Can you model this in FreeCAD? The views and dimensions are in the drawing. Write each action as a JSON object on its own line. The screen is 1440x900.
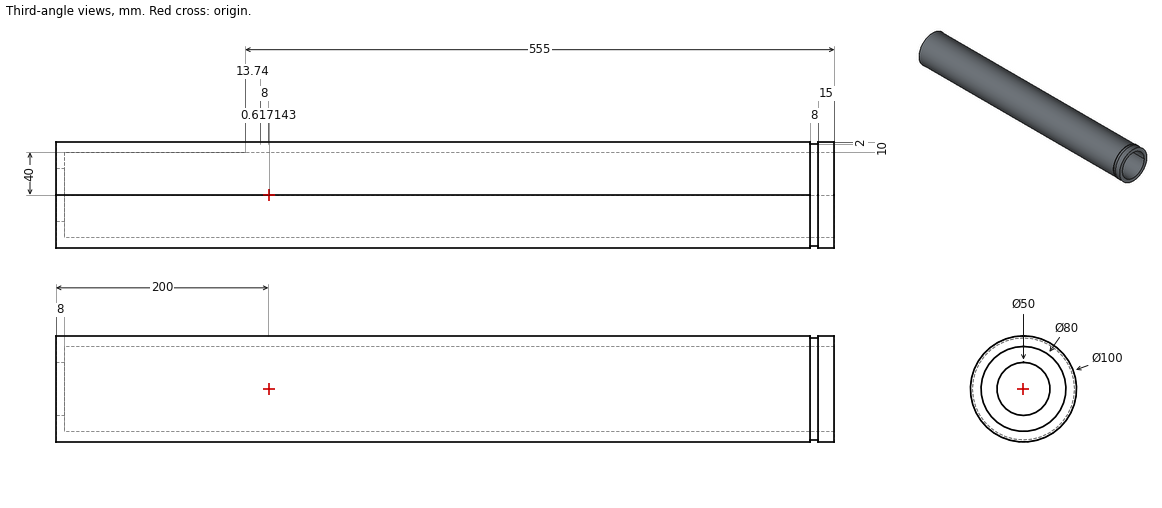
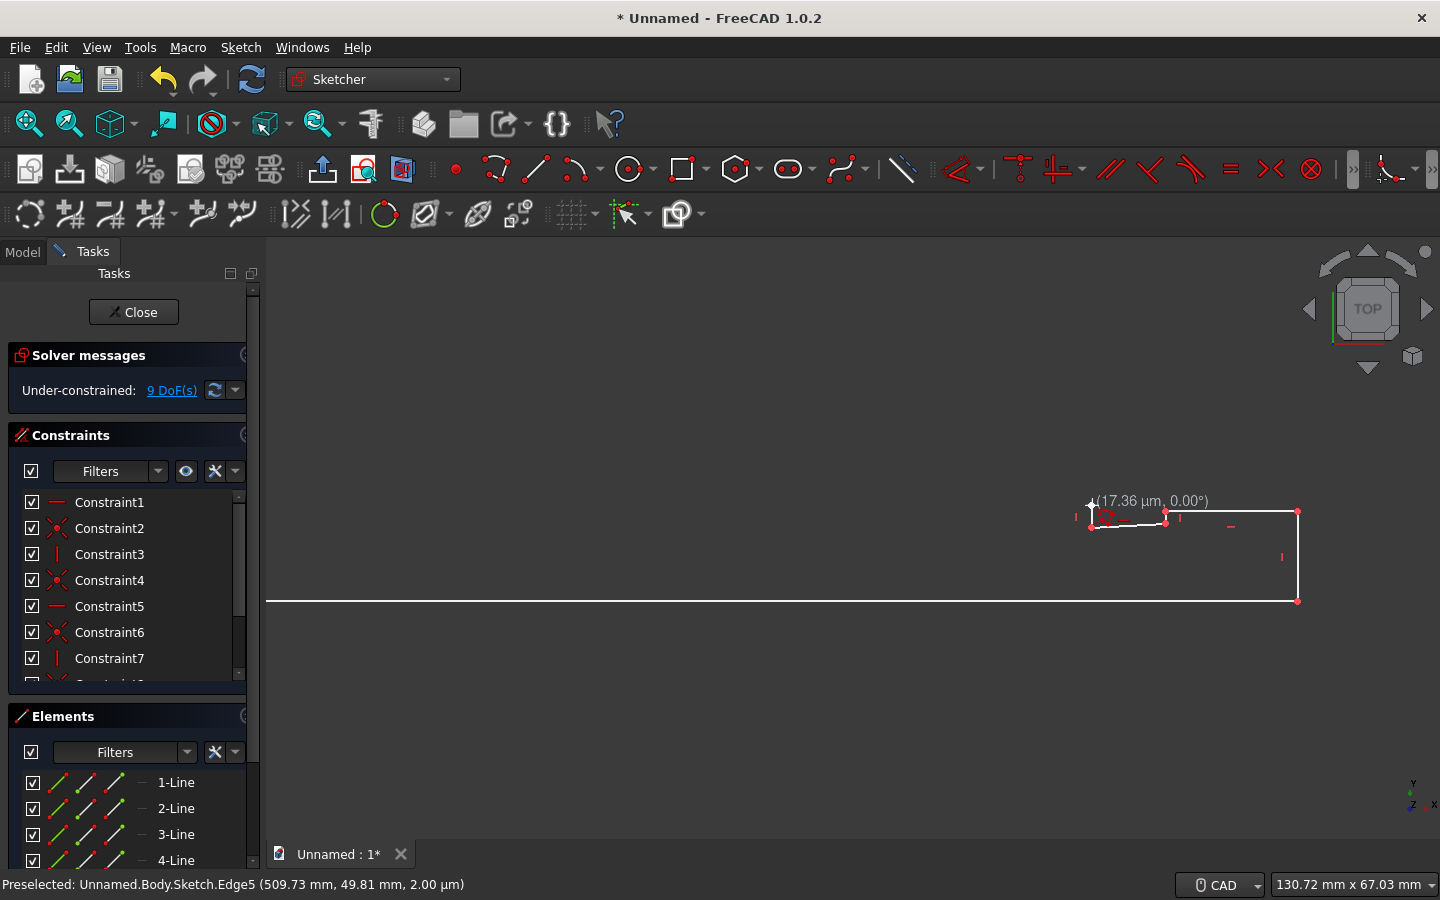
{"action": "scroll", "coordinate": [1094, 508], "scroll_direction": "down", "scroll_amount": 10}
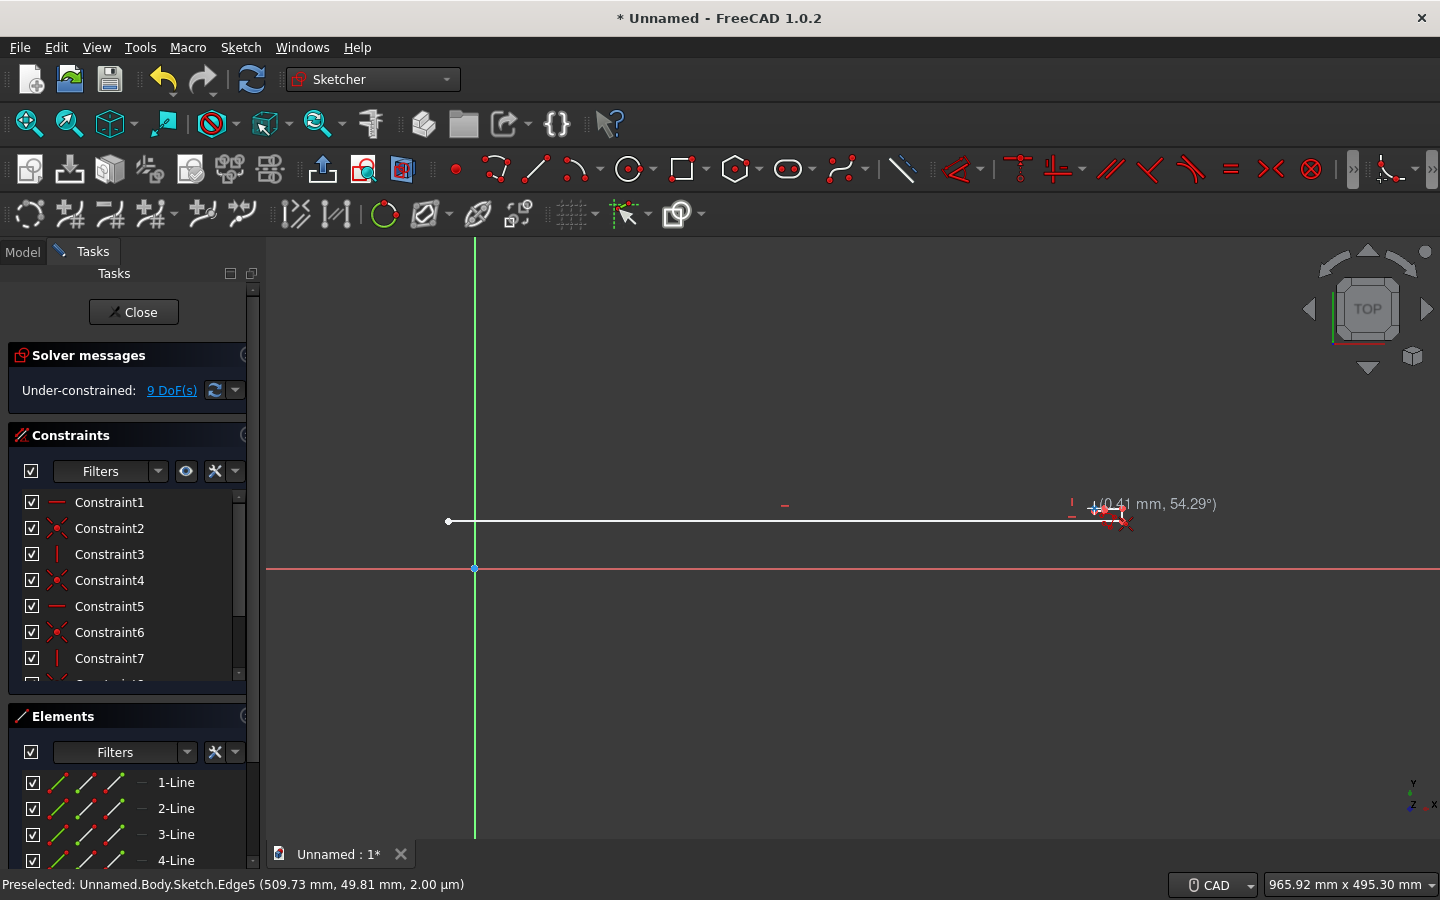
{"action": "scroll", "coordinate": [474, 508], "scroll_direction": "up", "scroll_amount": 16}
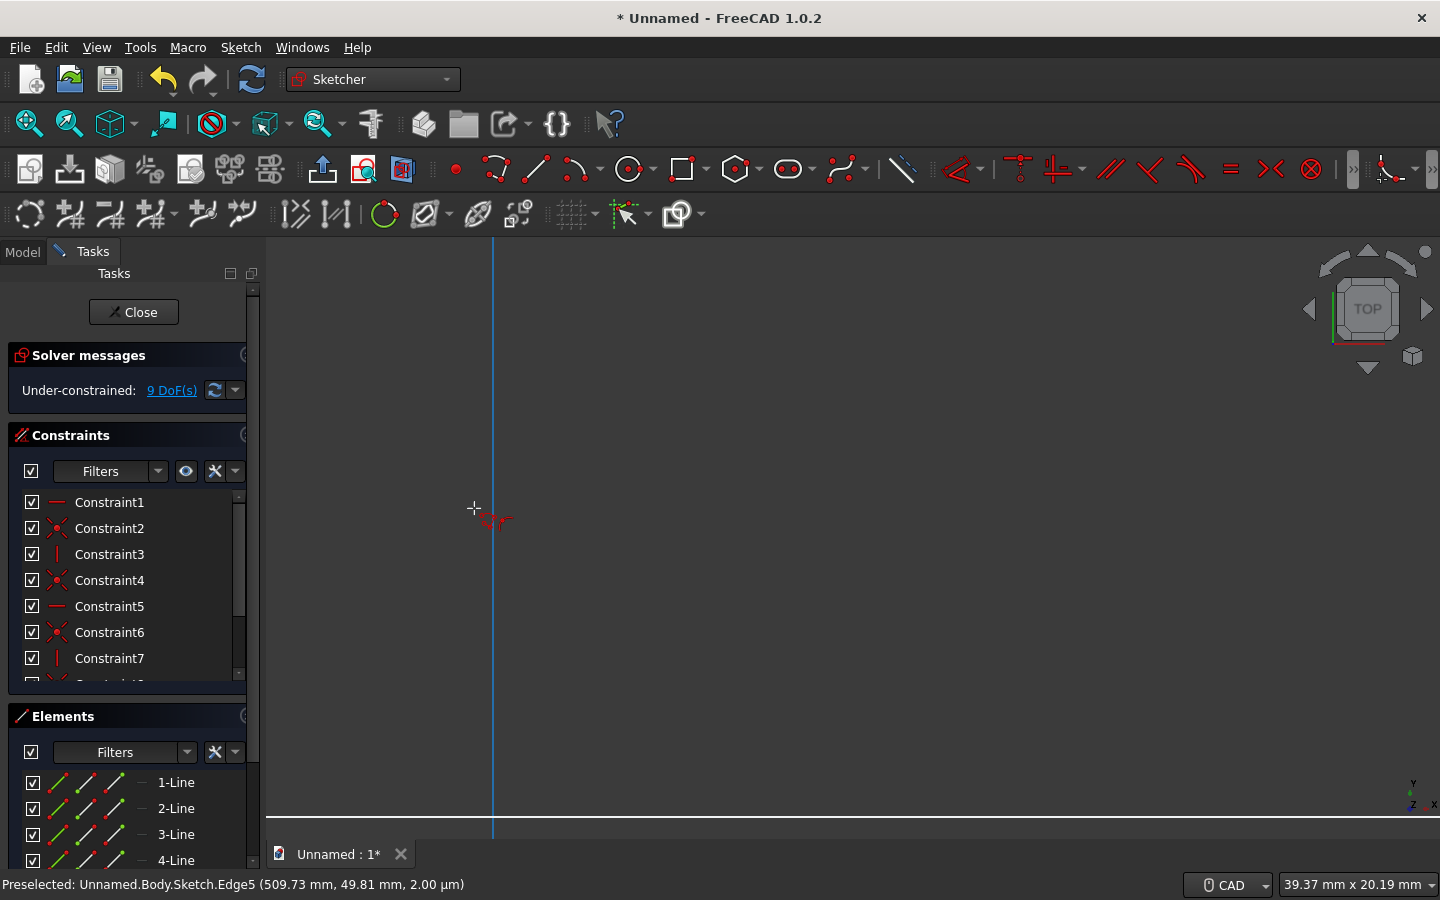
{"action": "left_click", "coordinate": [474, 497]}
{"action": "left_click", "coordinate": [474, 557]}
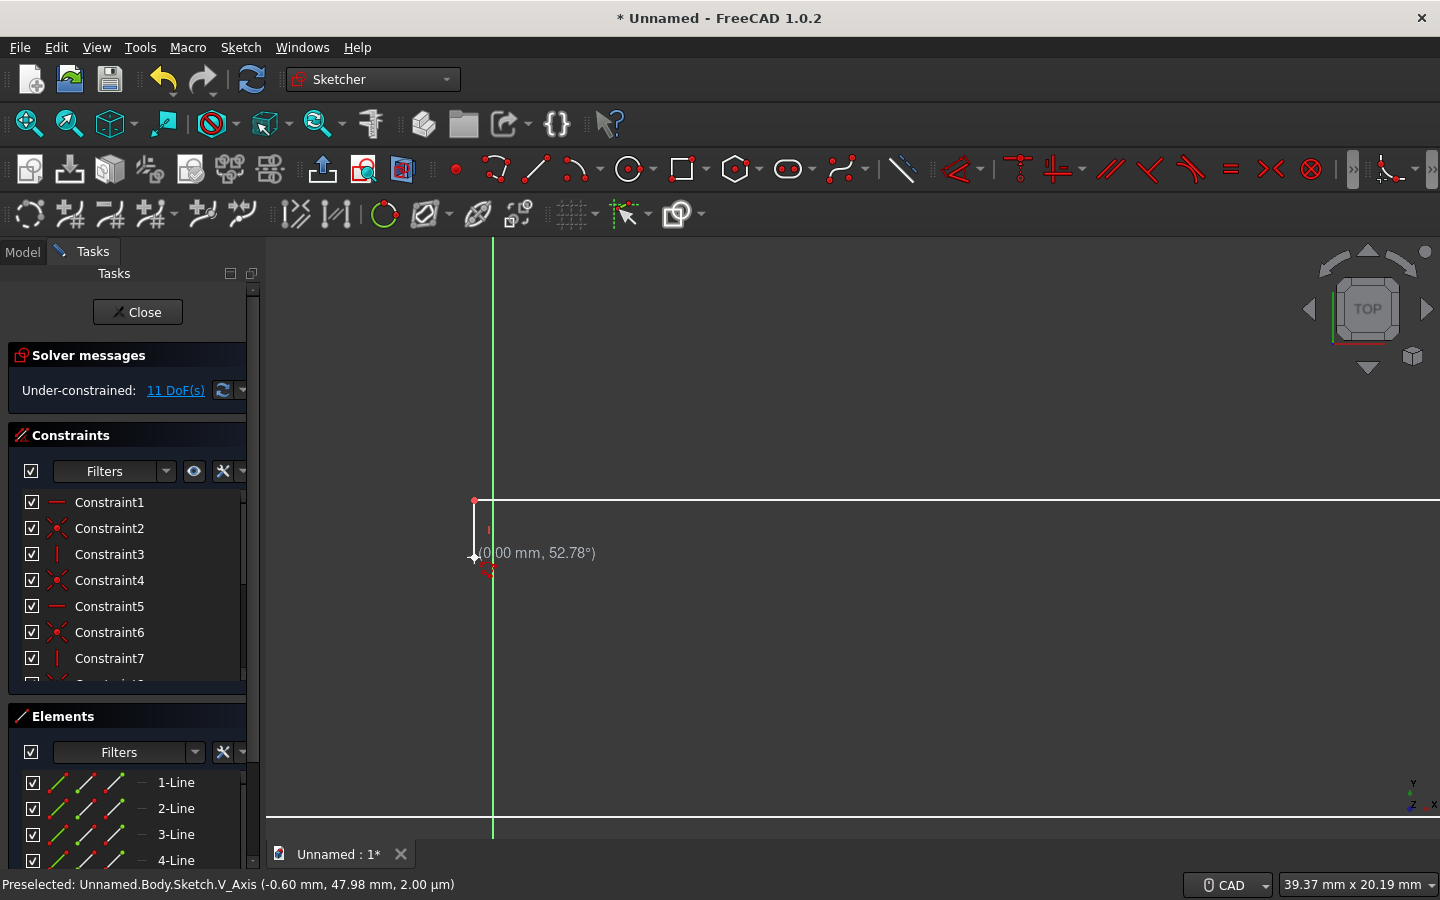
{"action": "scroll", "coordinate": [401, 501], "scroll_direction": "down", "scroll_amount": 15}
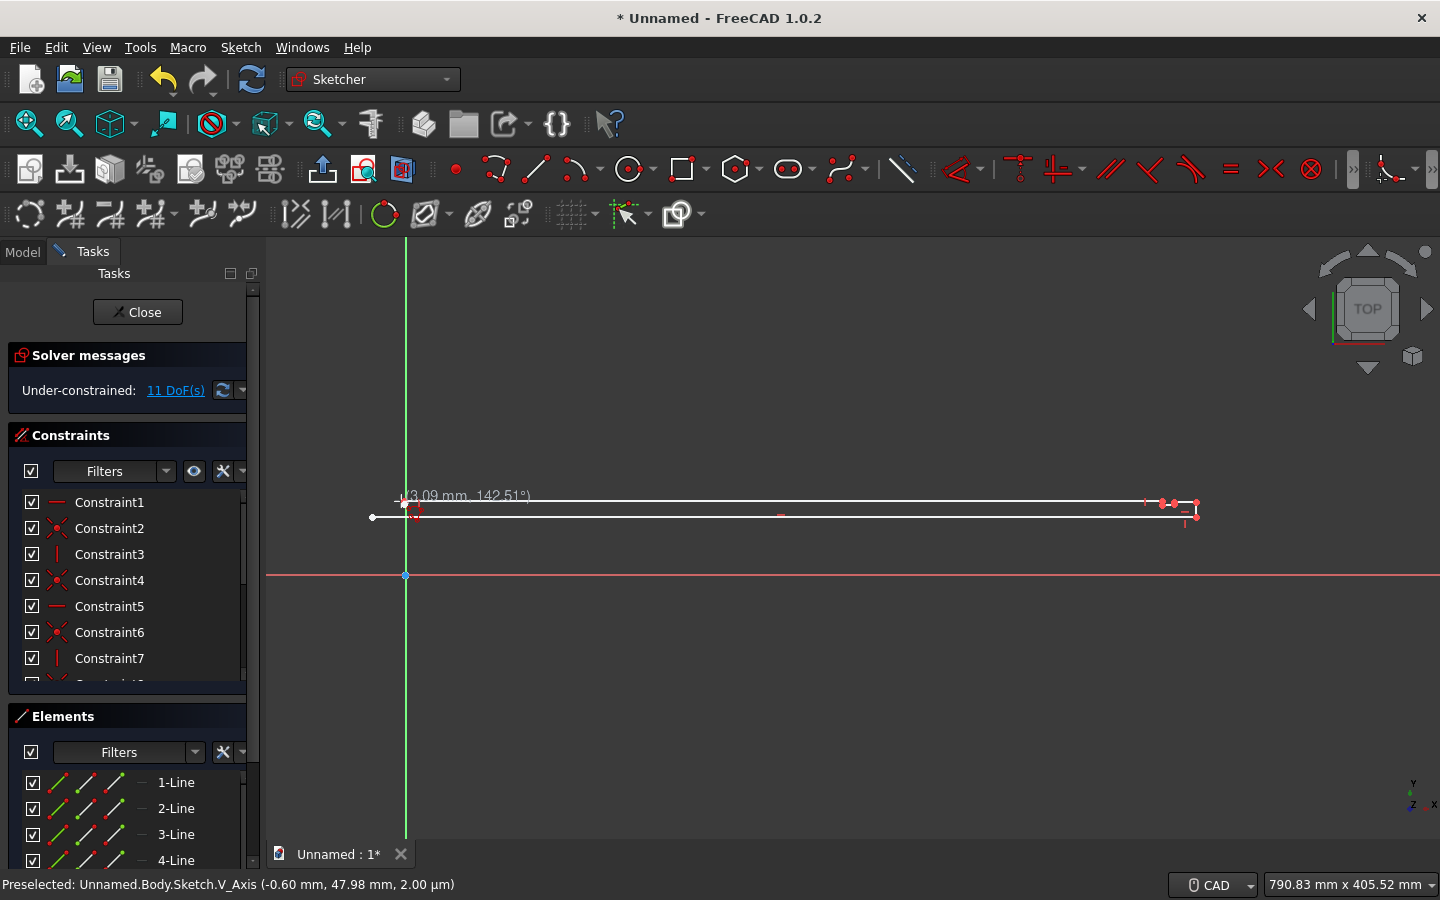
{"action": "scroll", "coordinate": [393, 504], "scroll_direction": "up", "scroll_amount": 2}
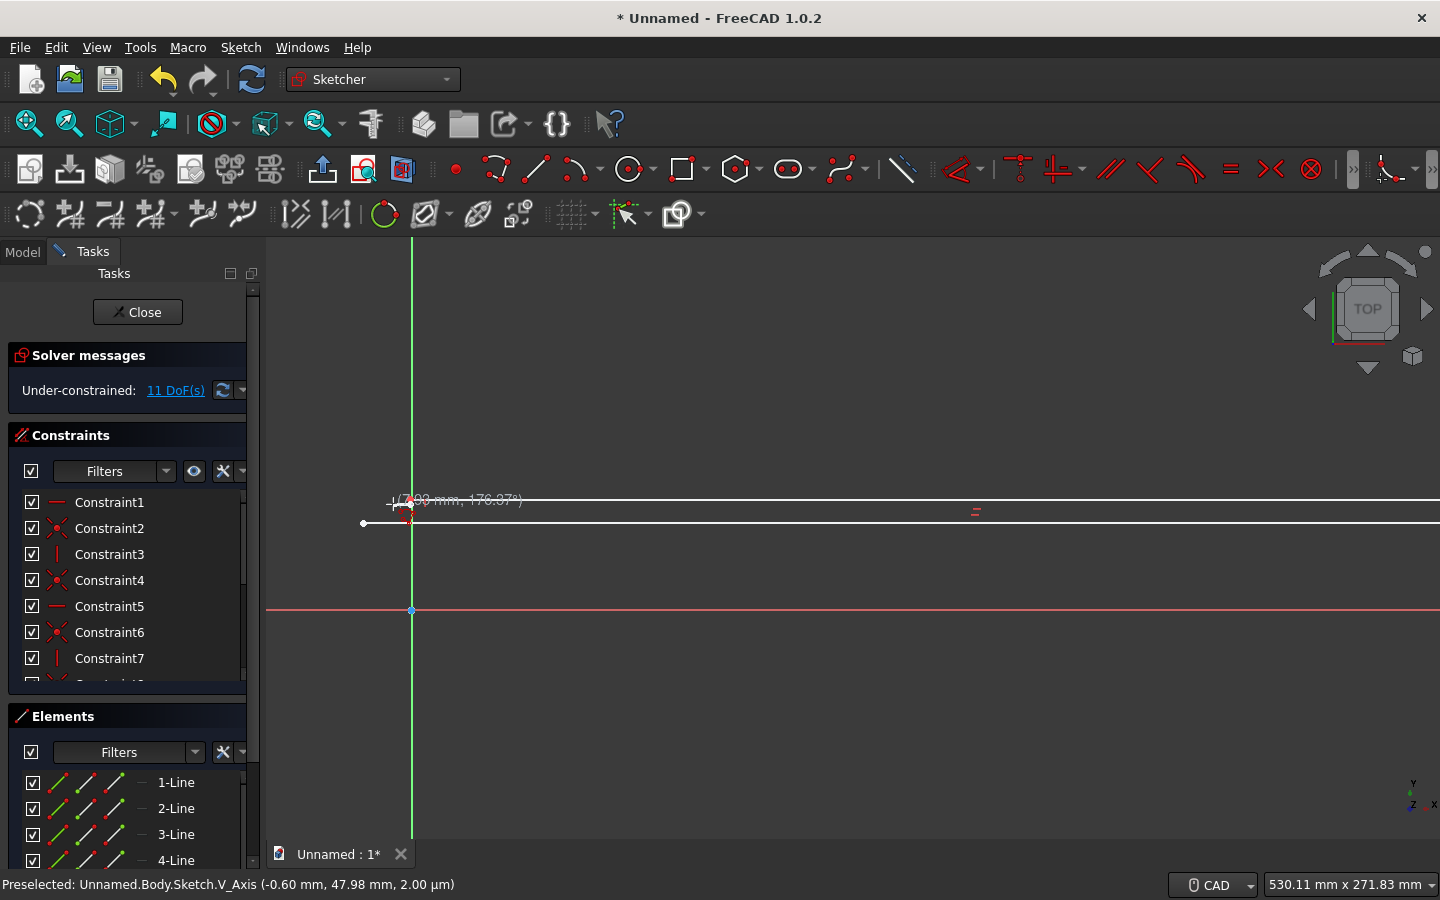
{"action": "left_click", "coordinate": [393, 504]}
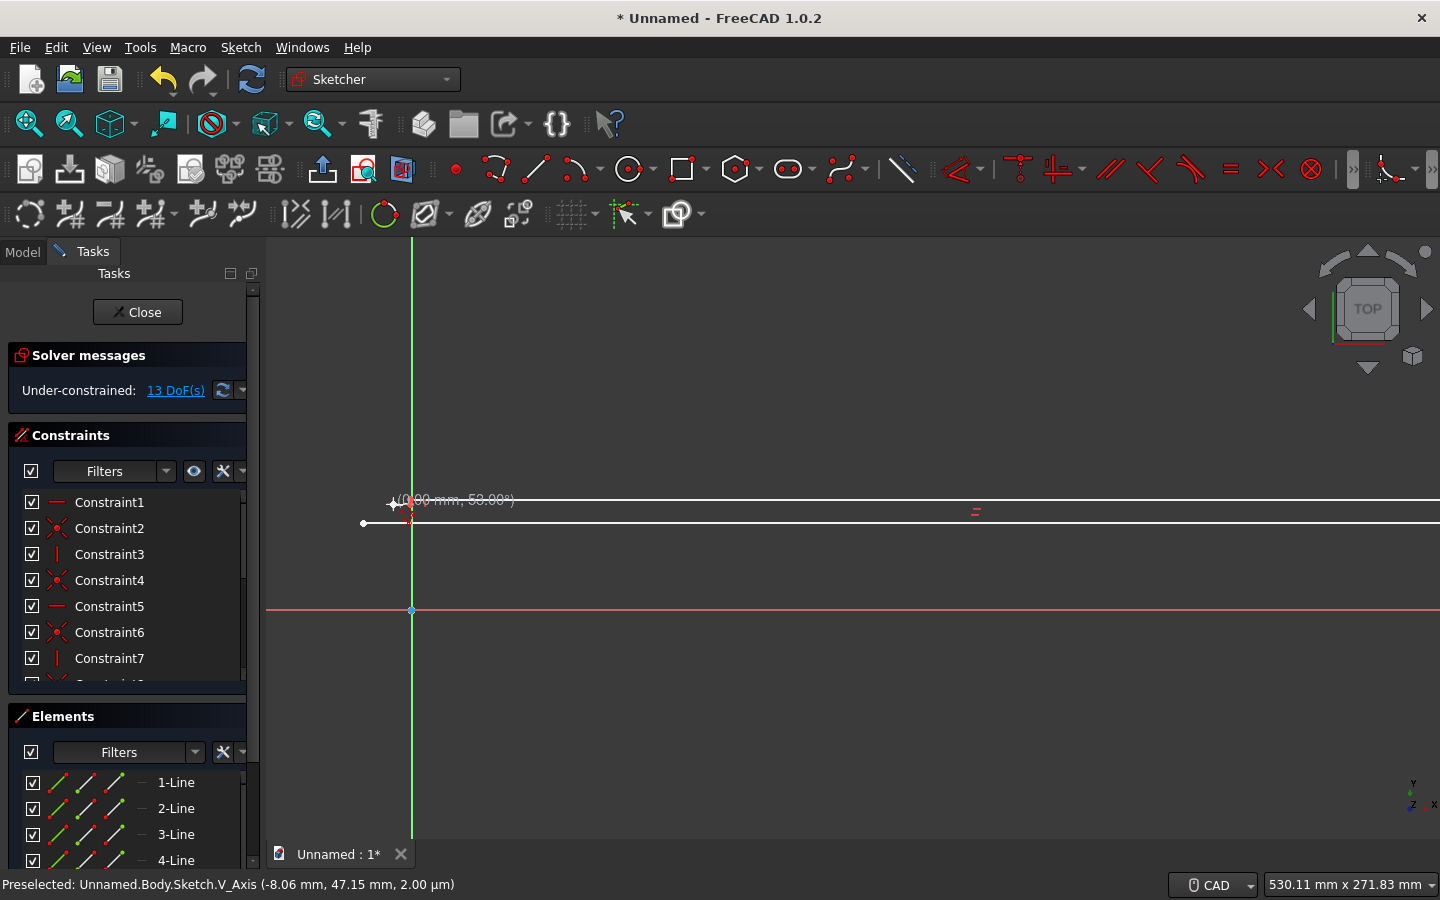
{"action": "scroll", "coordinate": [393, 500], "scroll_direction": "up", "scroll_amount": 7}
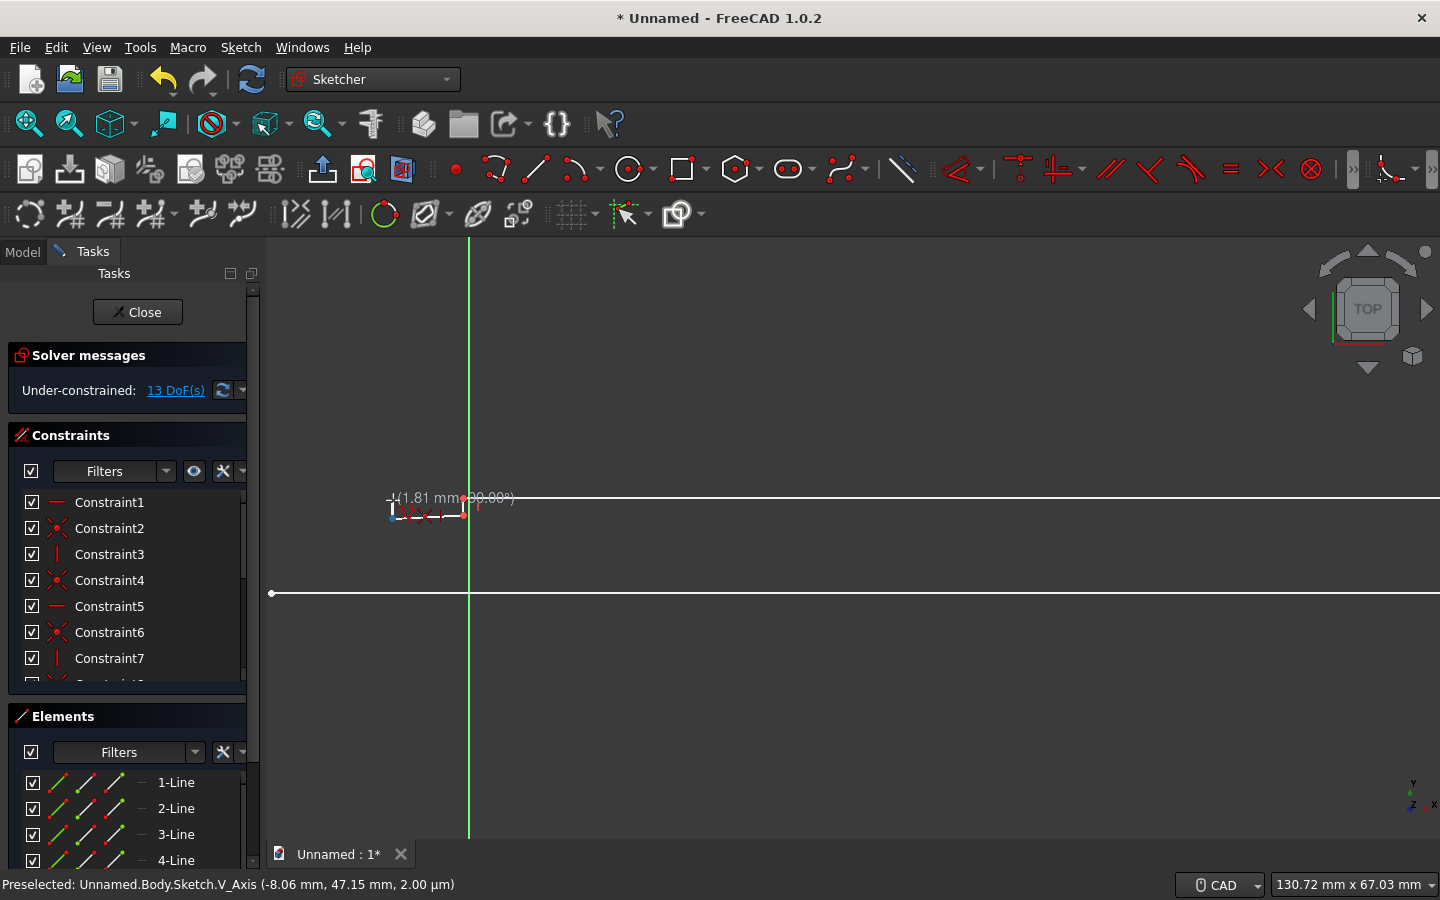
{"action": "left_click", "coordinate": [393, 497]}